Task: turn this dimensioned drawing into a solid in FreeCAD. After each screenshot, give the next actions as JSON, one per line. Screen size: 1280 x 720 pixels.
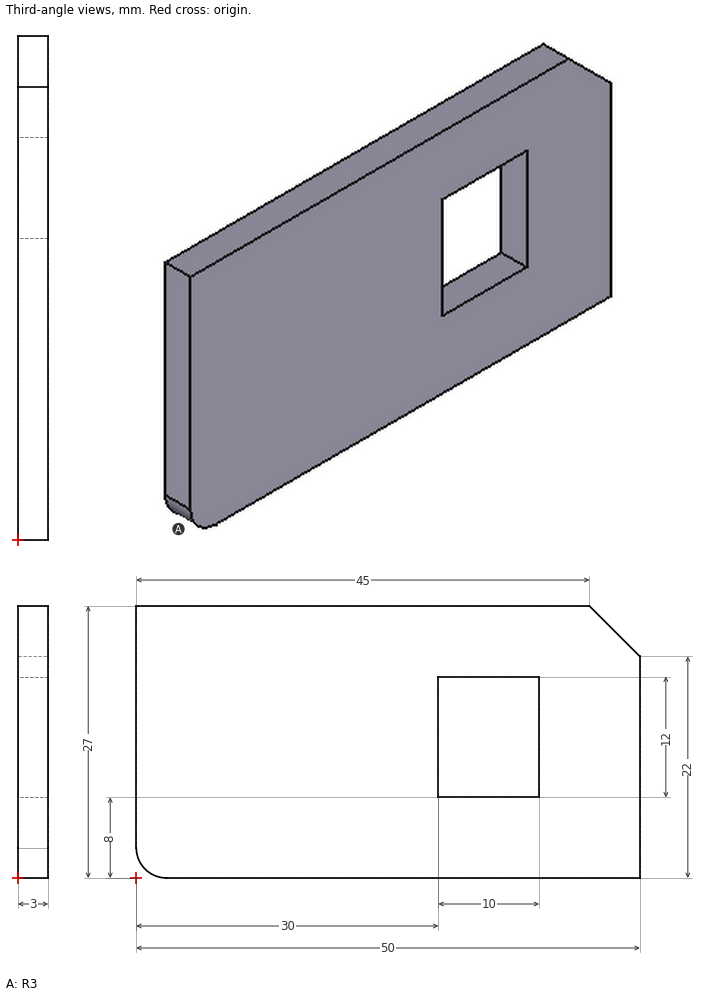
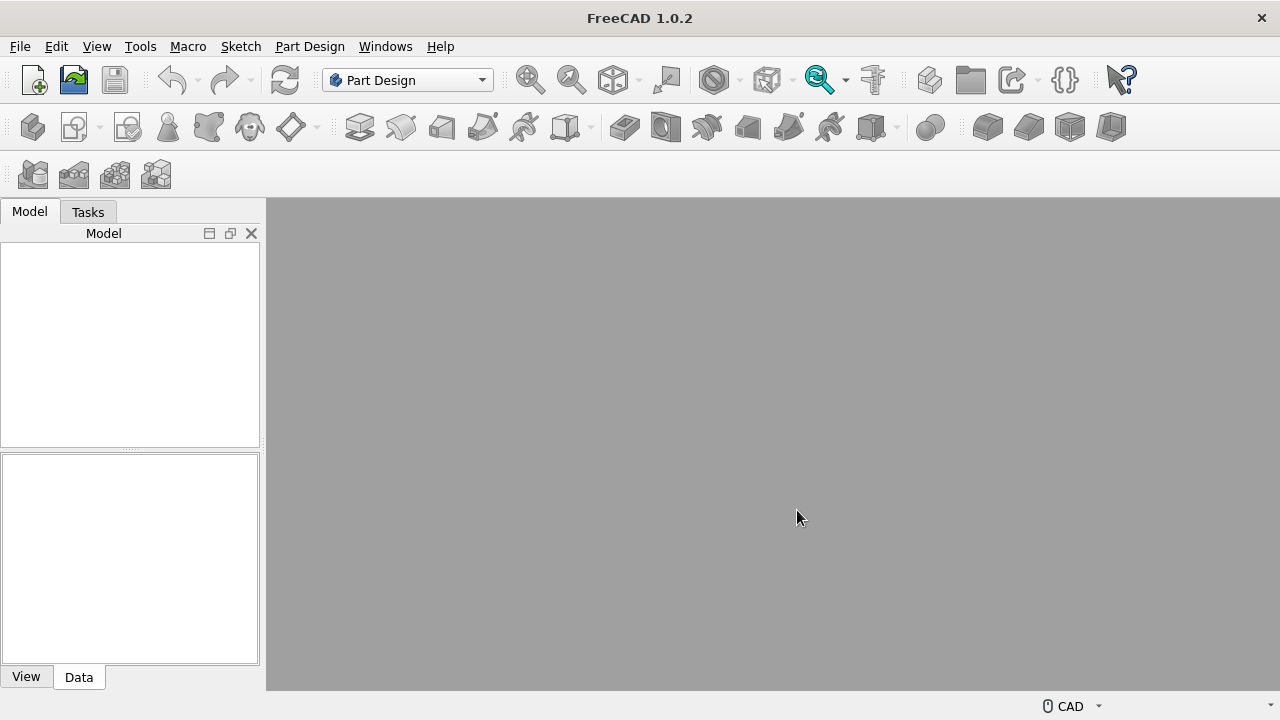
{"action": "left_click", "coordinate": [33, 80]}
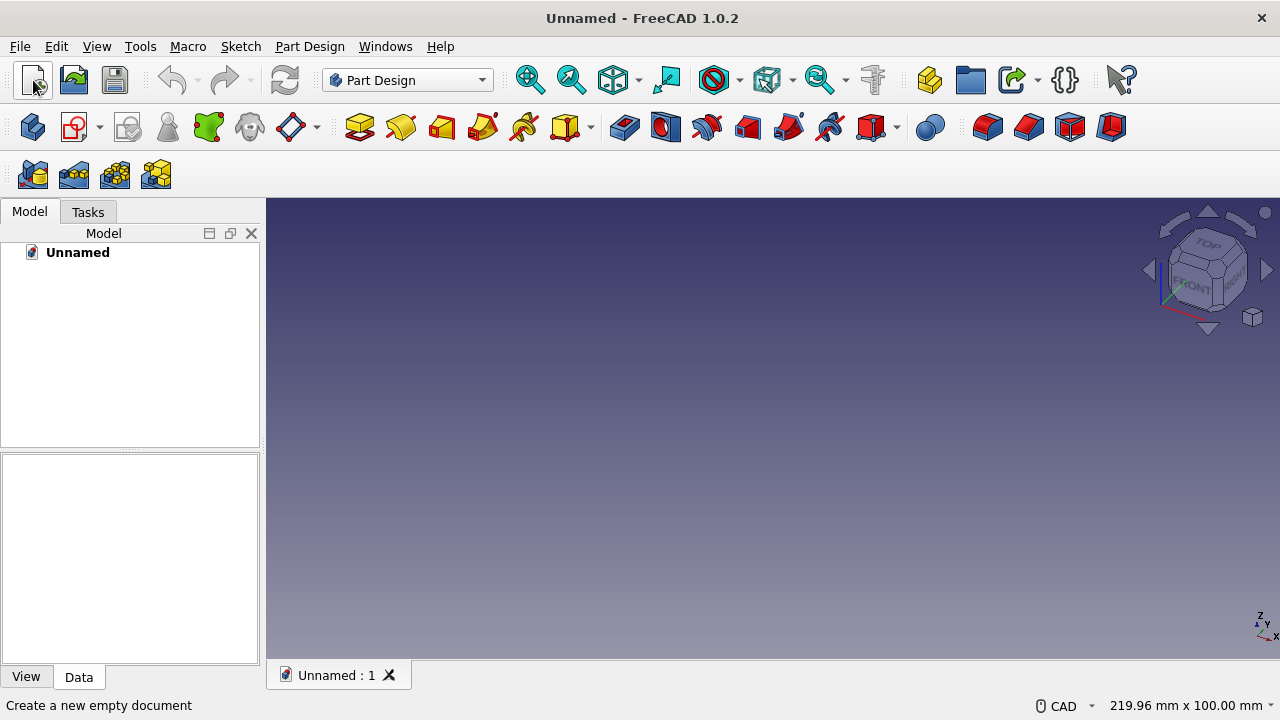
{"action": "left_click", "coordinate": [74, 128]}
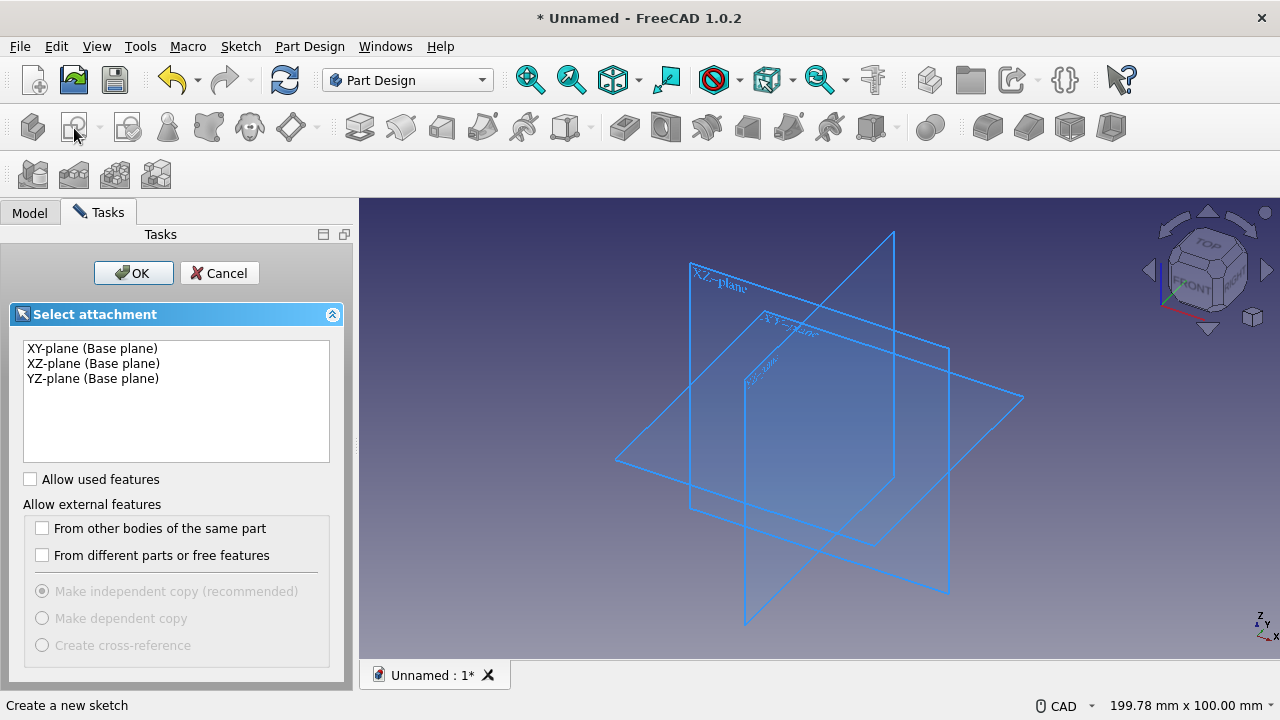
{"action": "left_click", "coordinate": [84, 378]}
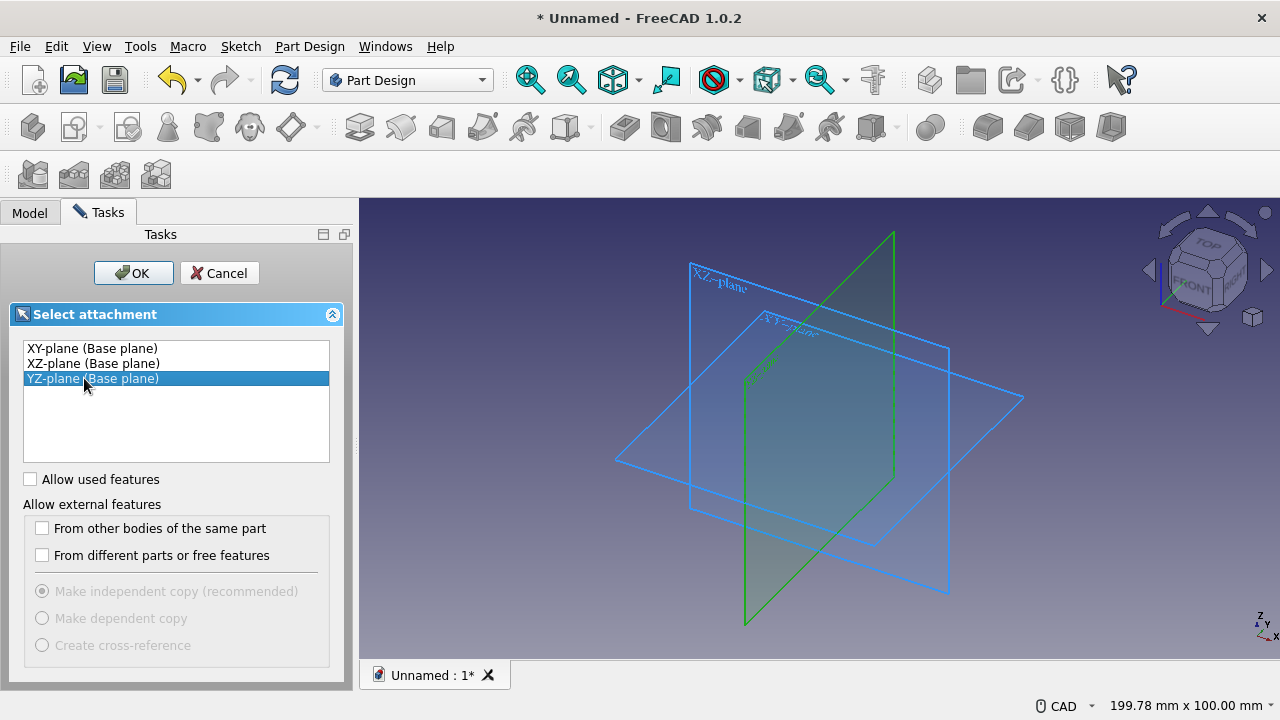
{"action": "left_click", "coordinate": [134, 273]}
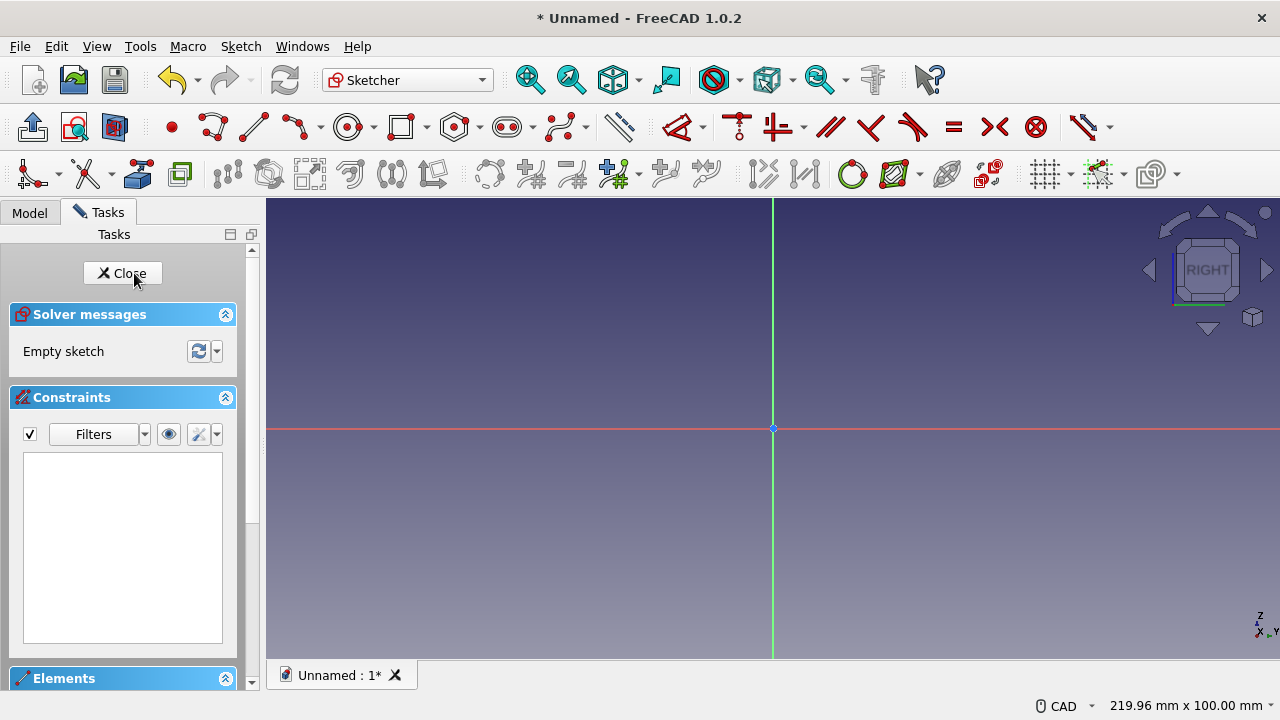
{"action": "scroll", "coordinate": [1038, 315], "scroll_direction": "up", "scroll_amount": 4}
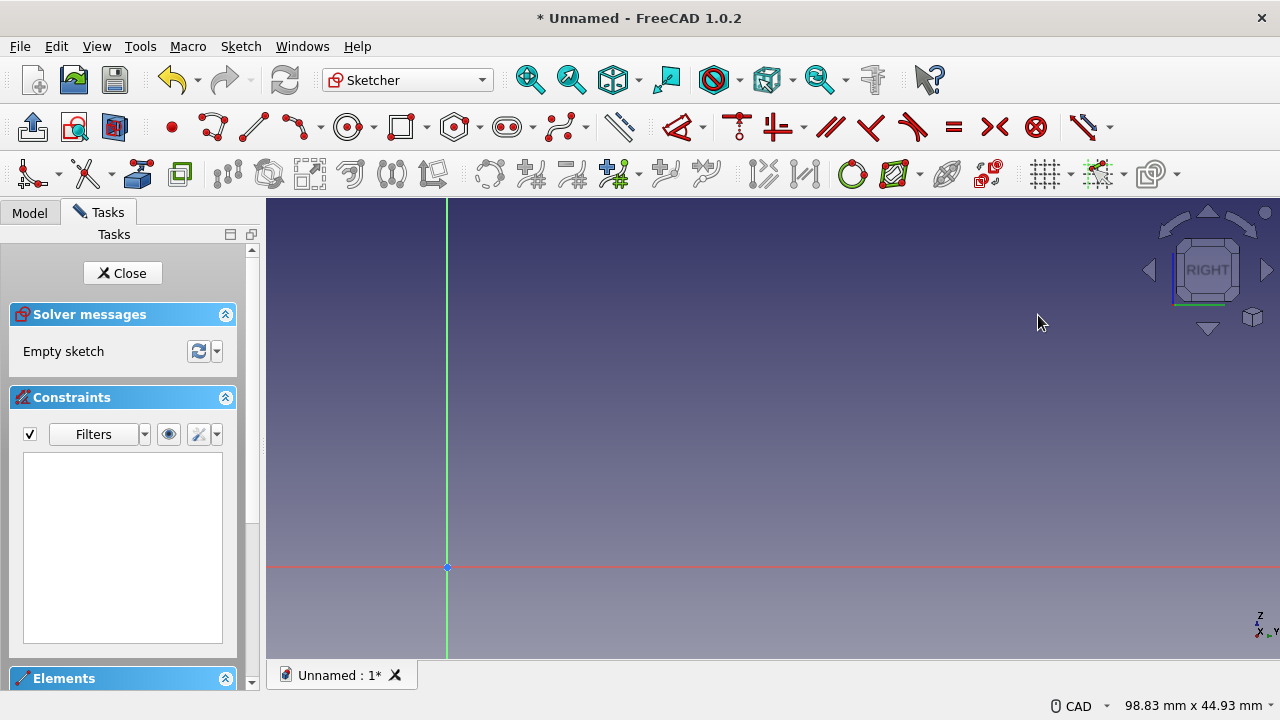
{"action": "left_click", "coordinate": [213, 128]}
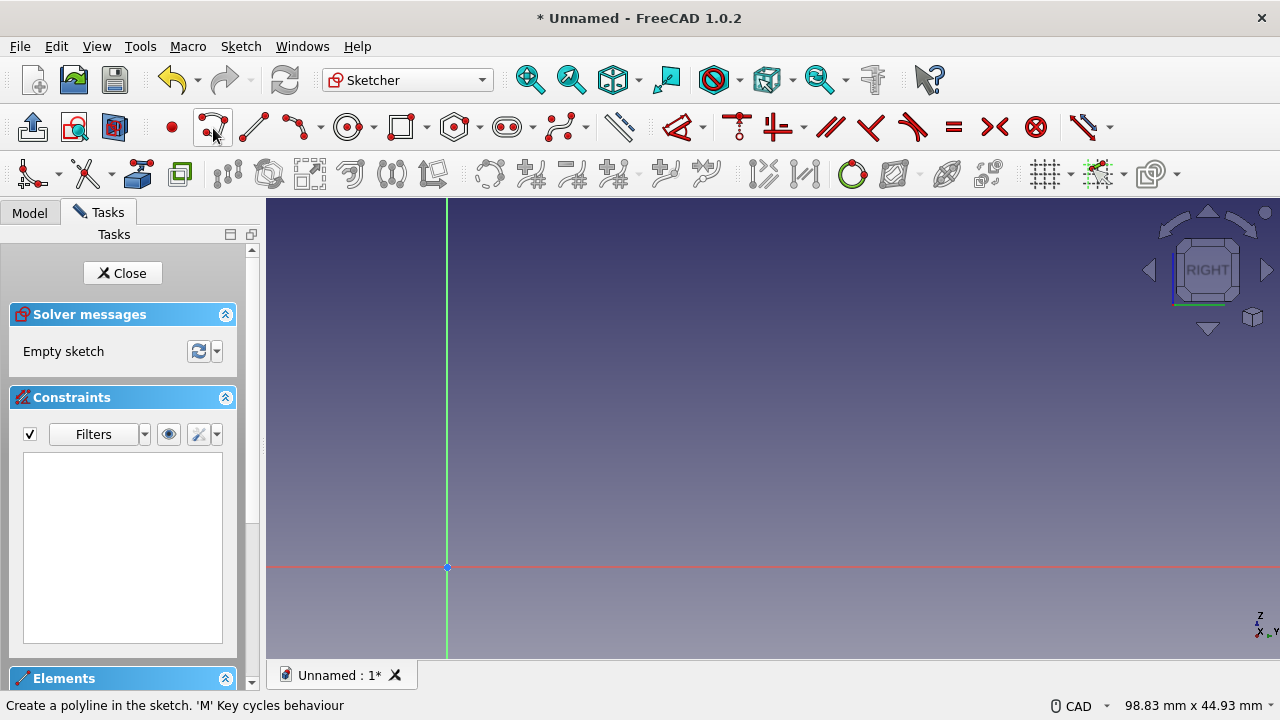
{"action": "left_click", "coordinate": [447, 567]}
{"action": "left_click", "coordinate": [960, 558]}
{"action": "left_click", "coordinate": [960, 342]}
{"action": "left_click", "coordinate": [909, 290]}
{"action": "left_click", "coordinate": [456, 290]}
{"action": "left_click", "coordinate": [447, 567]}
{"action": "key", "text": "Escape"}
{"action": "key", "text": "Escape"}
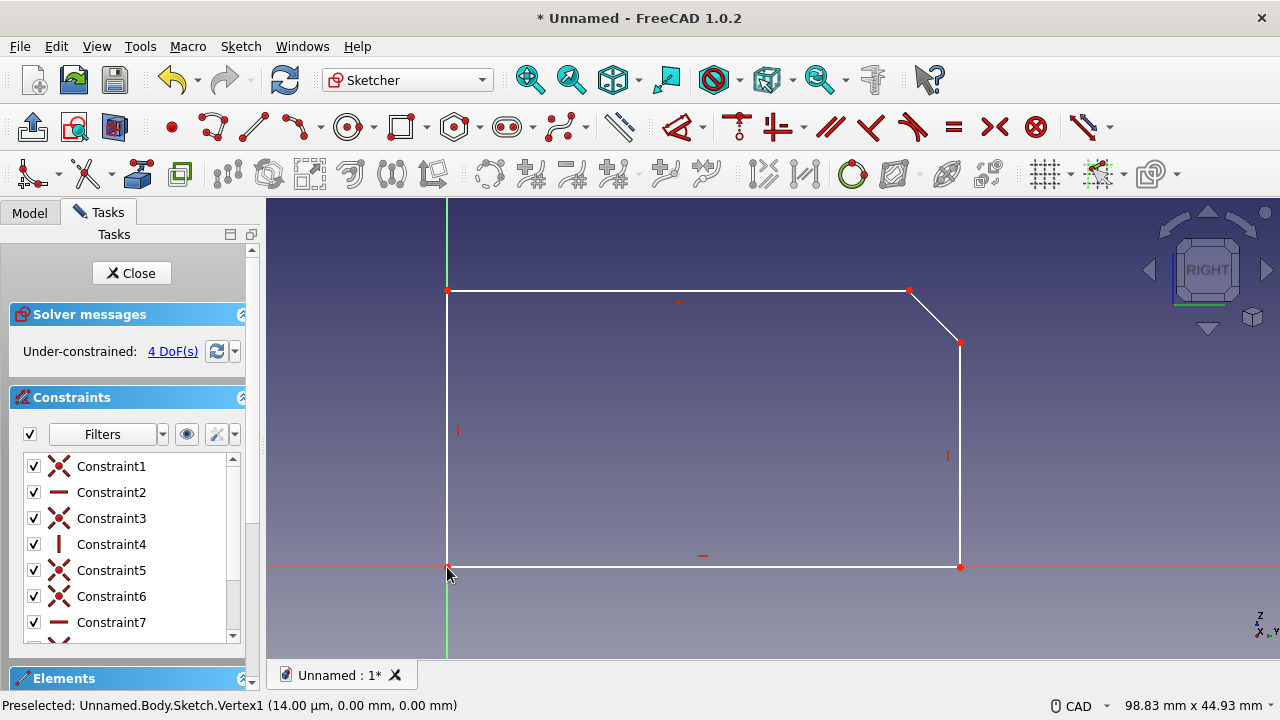
{"action": "left_click", "coordinate": [676, 128]}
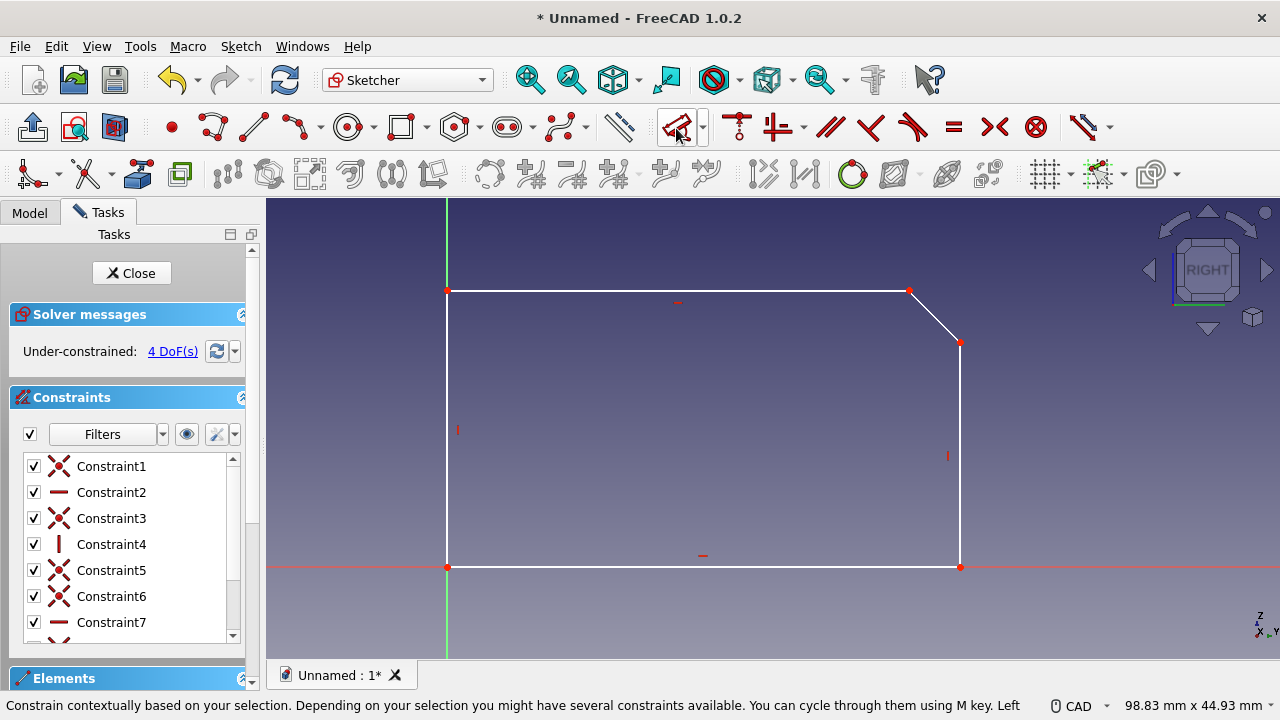
{"action": "left_click", "coordinate": [601, 567]}
{"action": "left_click", "coordinate": [704, 601]}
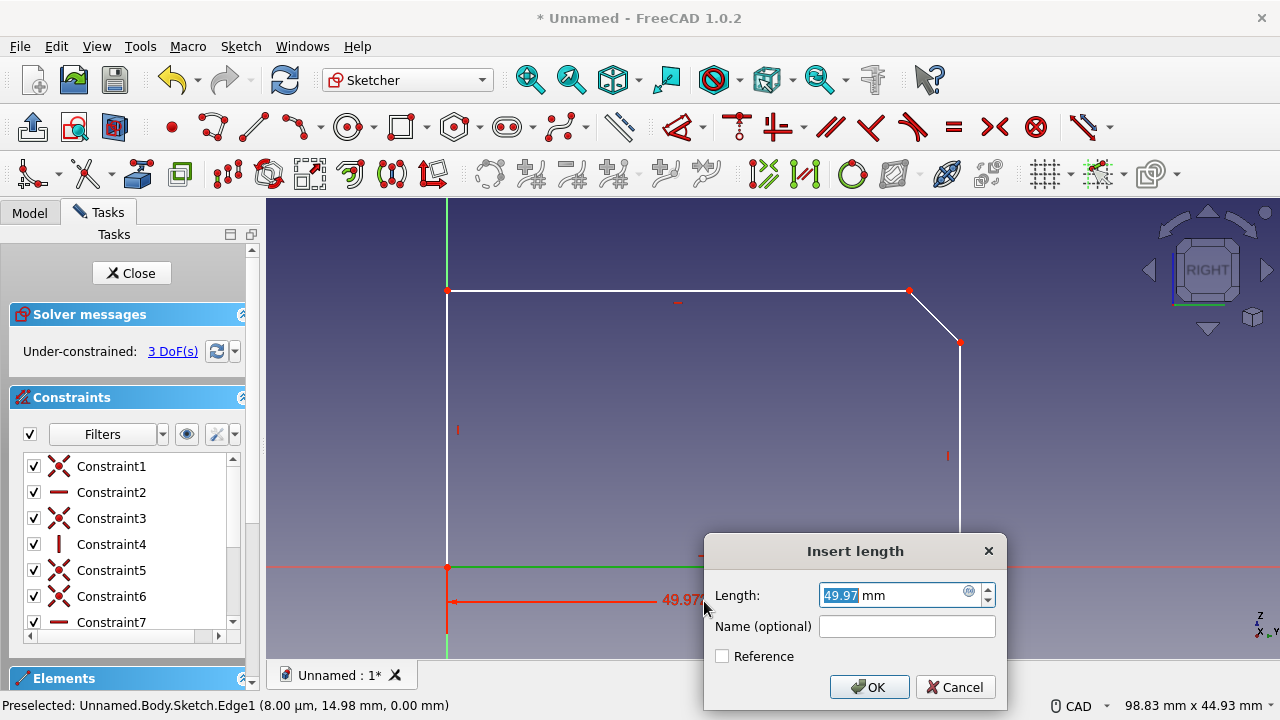
{"action": "type", "text": "50"}
{"action": "key", "text": "Return"}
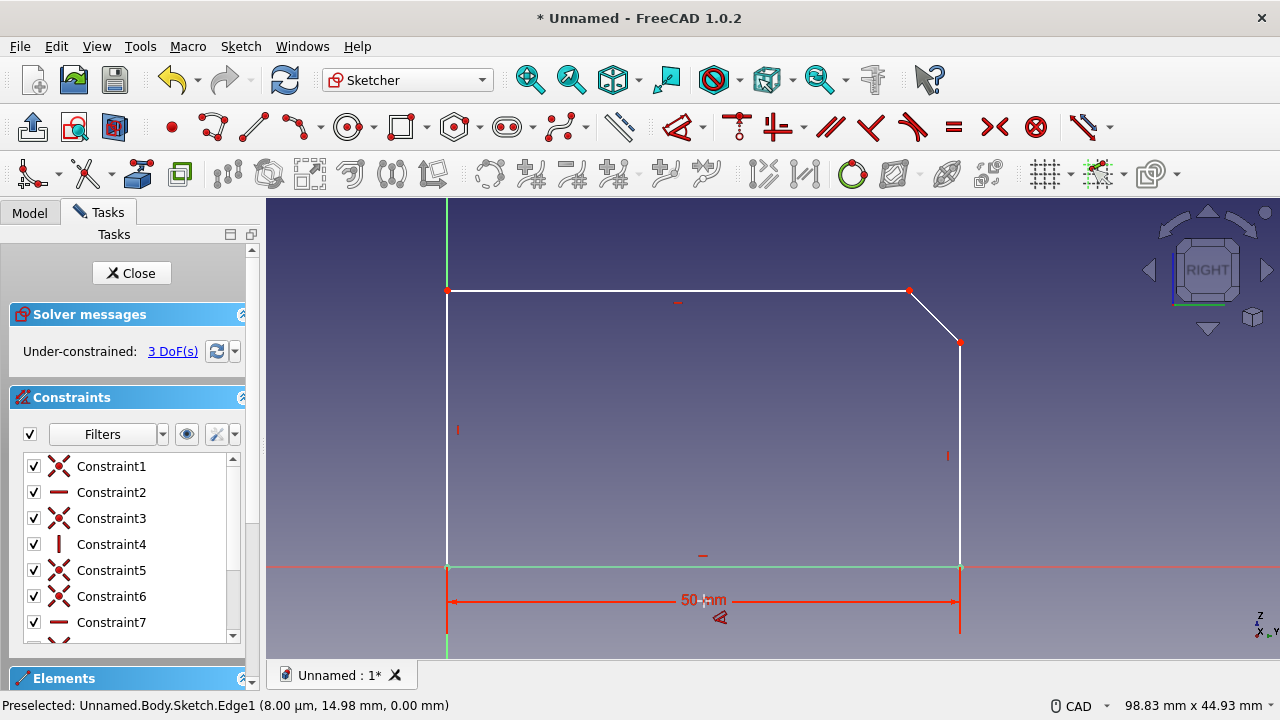
{"action": "left_click", "coordinate": [960, 500]}
{"action": "left_click", "coordinate": [994, 455]}